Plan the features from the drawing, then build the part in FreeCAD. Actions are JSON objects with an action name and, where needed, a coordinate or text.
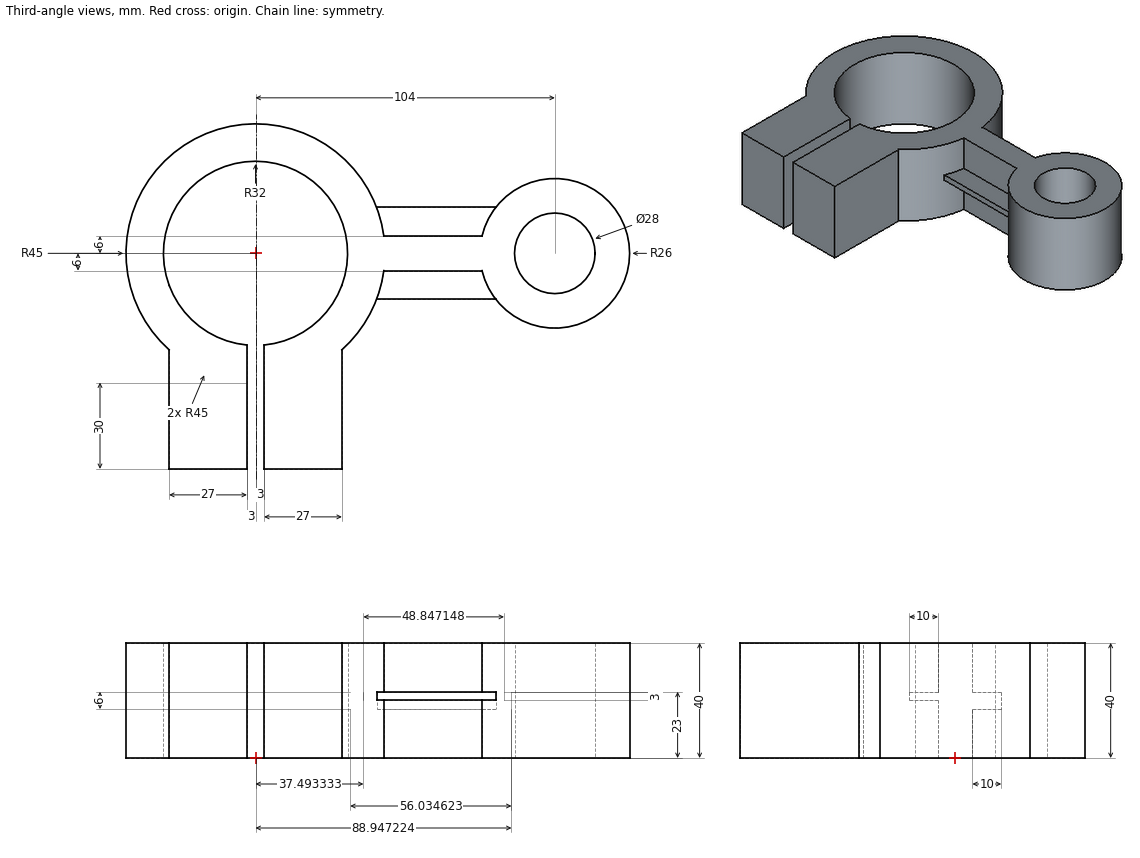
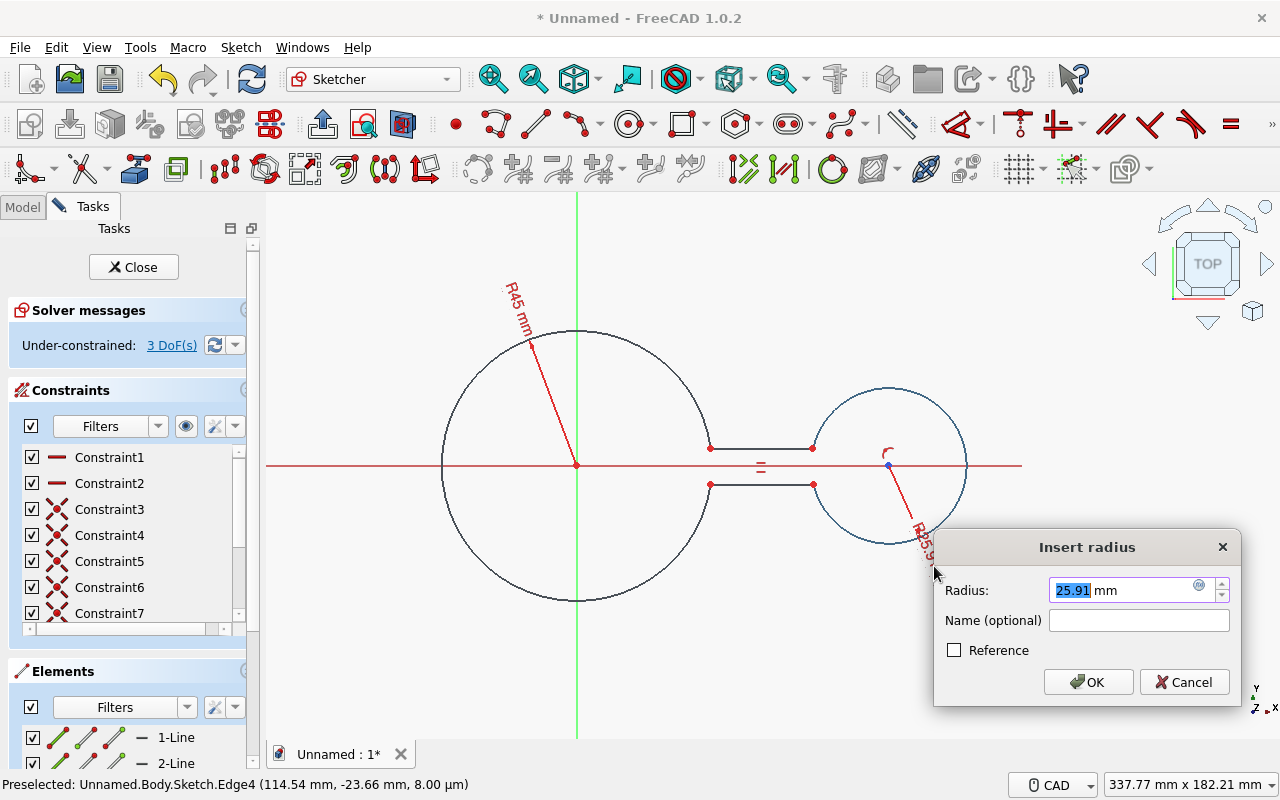
{"action": "type", "text": "26"}
{"action": "key", "text": "Return"}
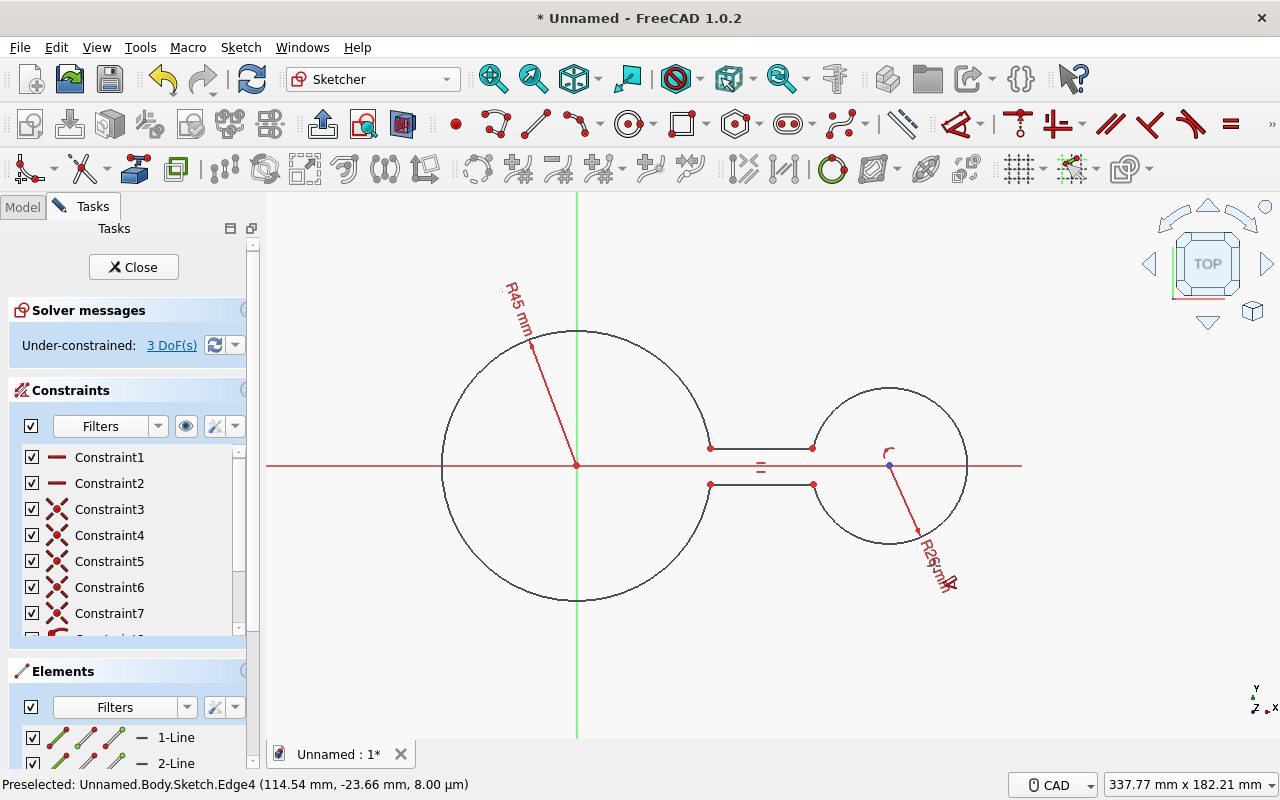
{"action": "scroll", "coordinate": [813, 449], "scroll_direction": "up", "scroll_amount": 4}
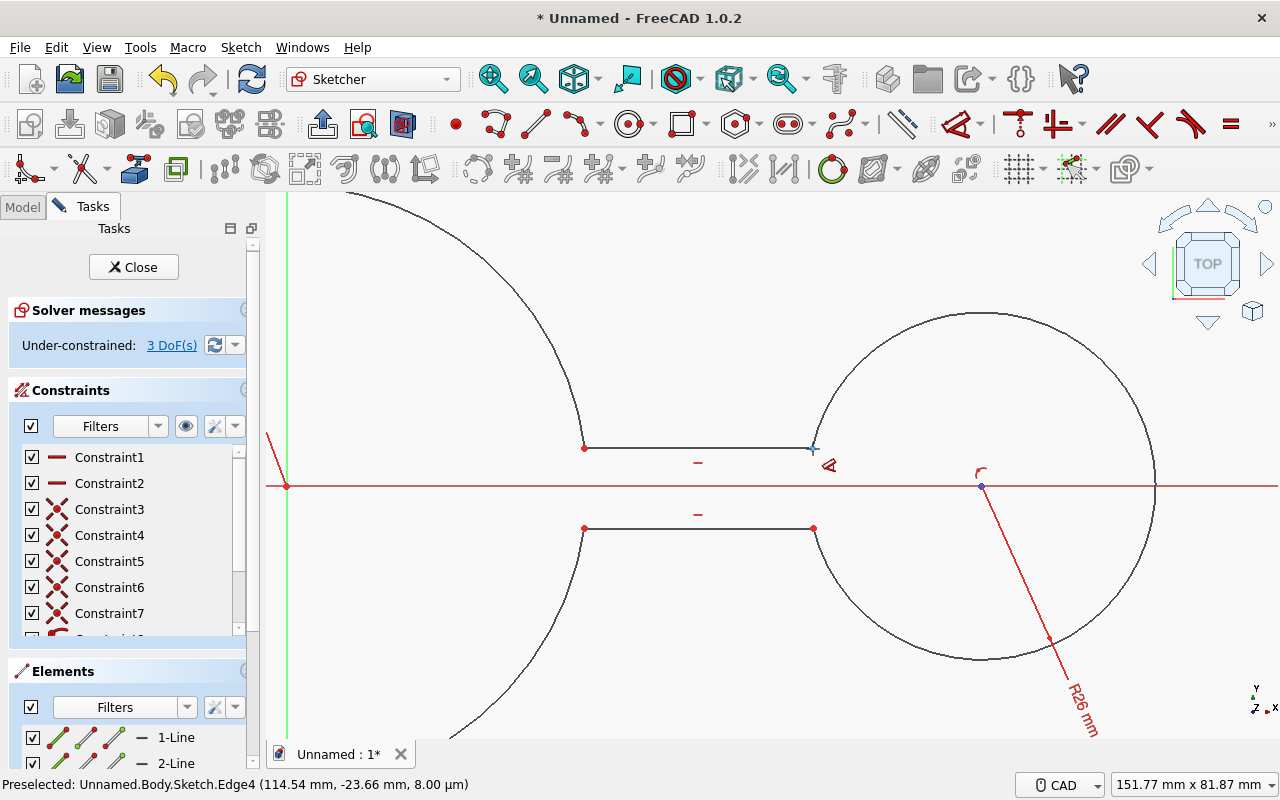
{"action": "left_click", "coordinate": [812, 448]}
{"action": "left_click", "coordinate": [846, 467]}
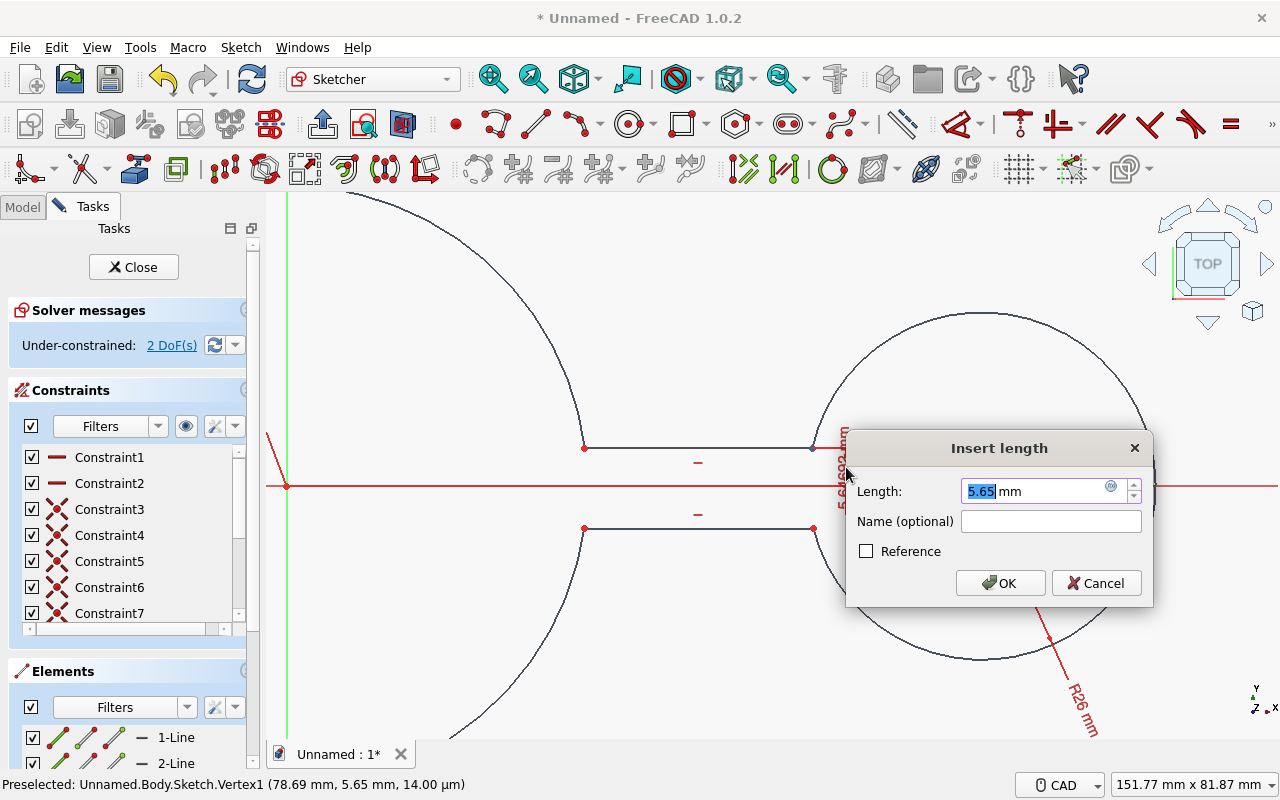
{"action": "type", "text": "6"}
{"action": "key", "text": "Return"}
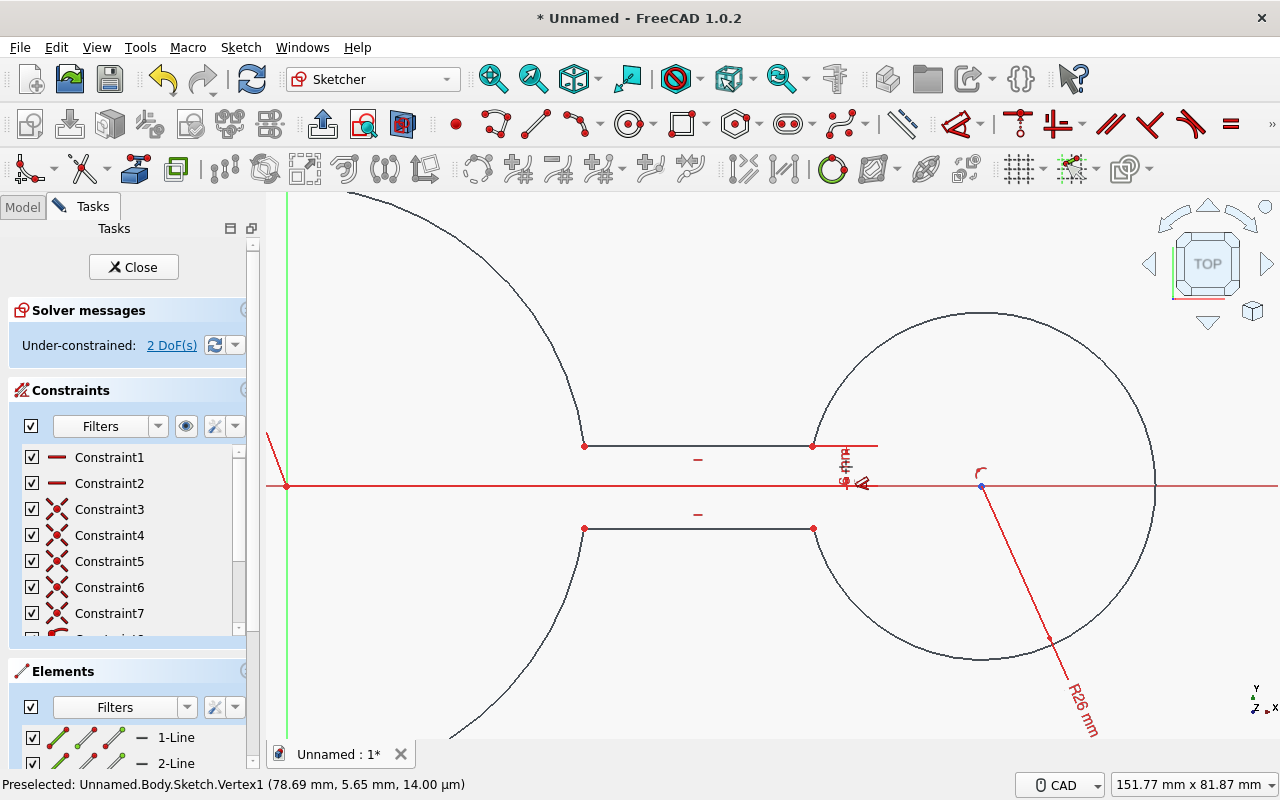
{"action": "left_click", "coordinate": [584, 529]}
{"action": "left_click", "coordinate": [618, 507]}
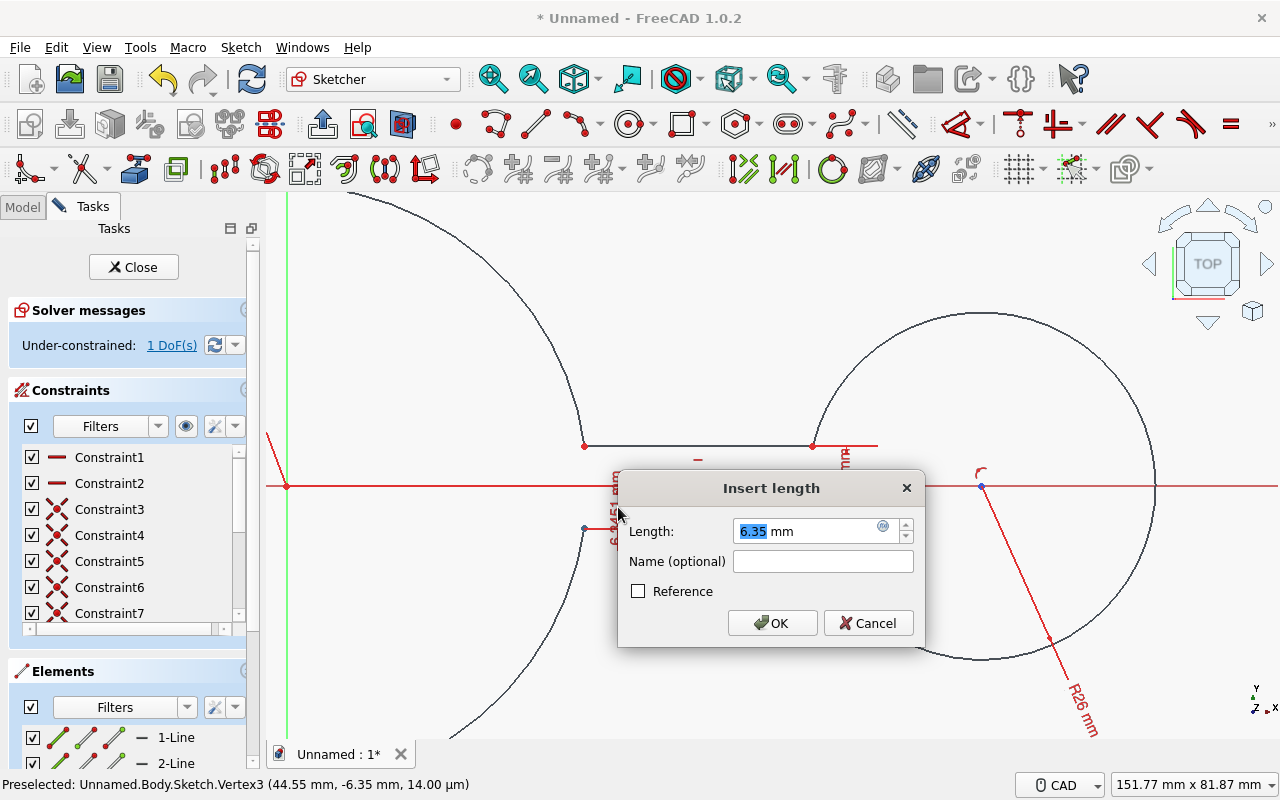
{"action": "type", "text": "6"}
{"action": "key", "text": "Return"}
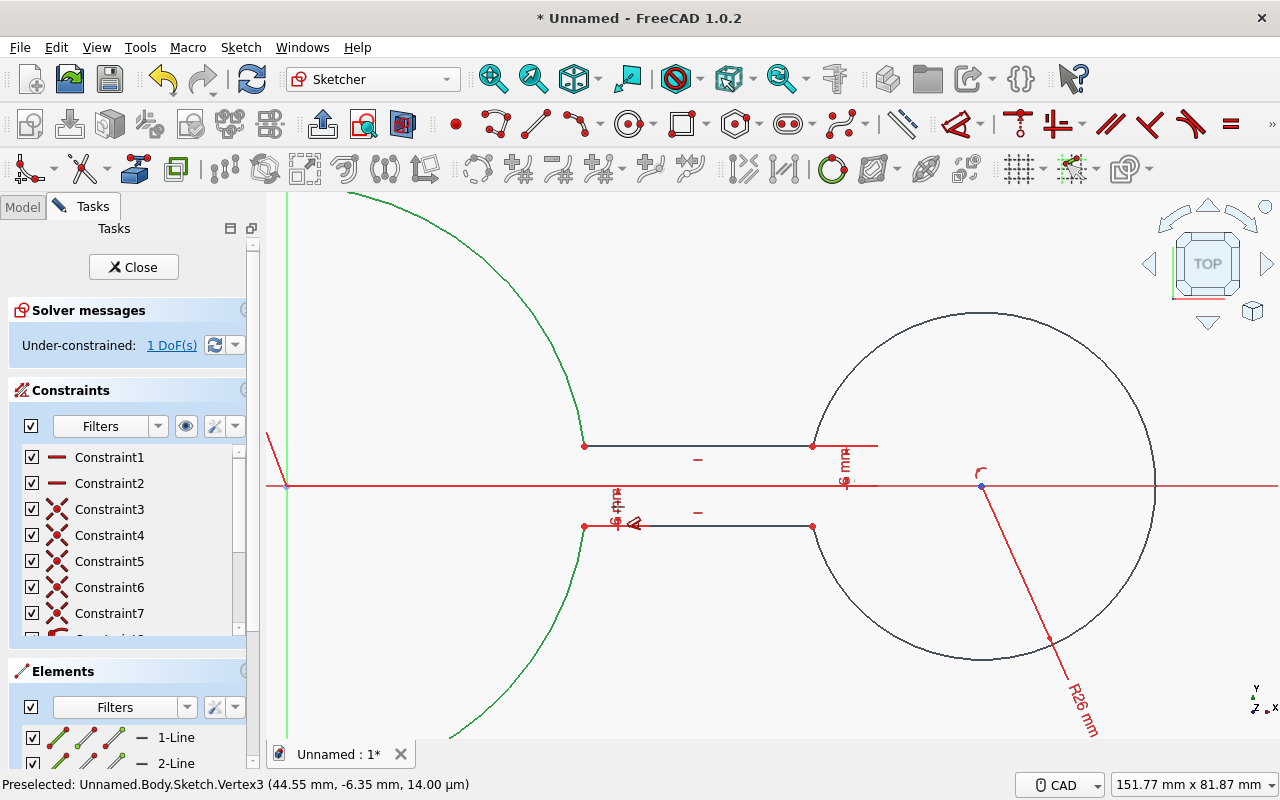
{"action": "left_click", "coordinate": [982, 486]}
{"action": "left_click", "coordinate": [480, 520]}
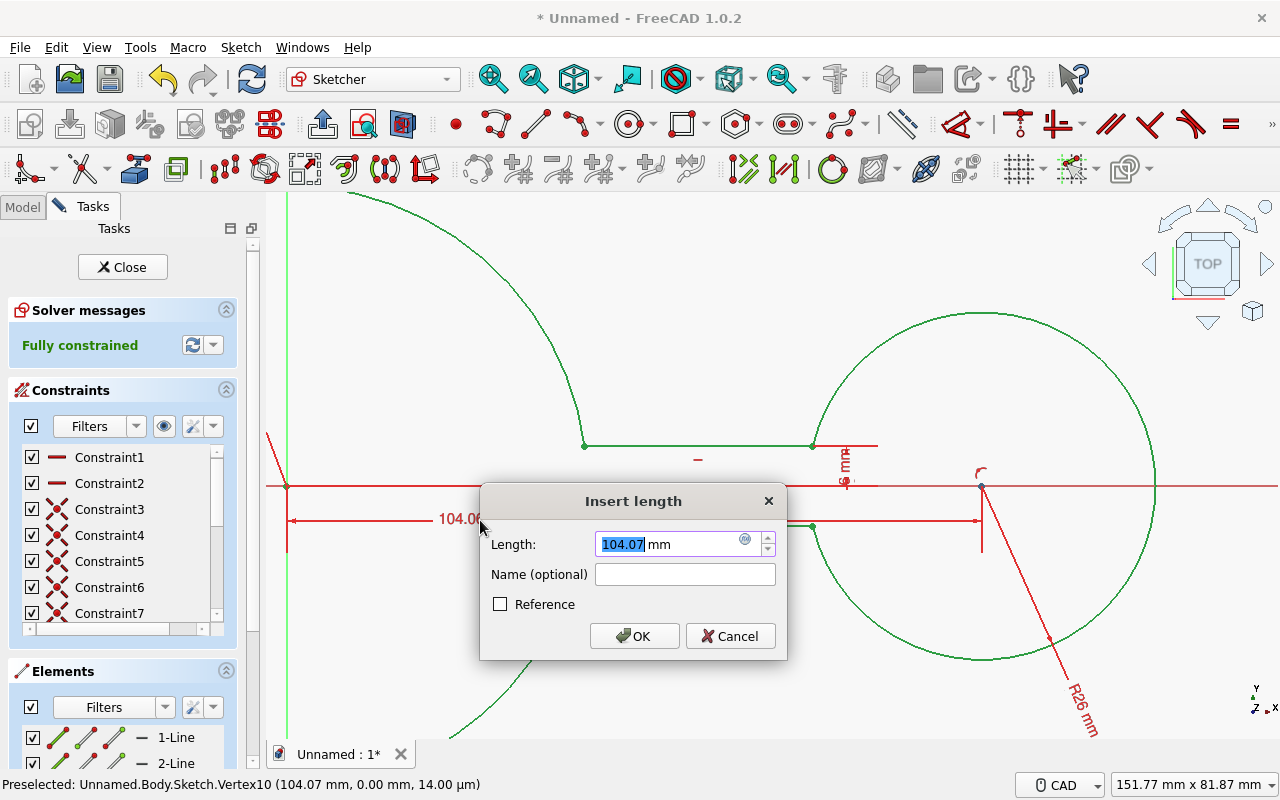
{"action": "type", "text": "104"}
{"action": "key", "text": "Return"}
{"action": "key", "text": "Escape"}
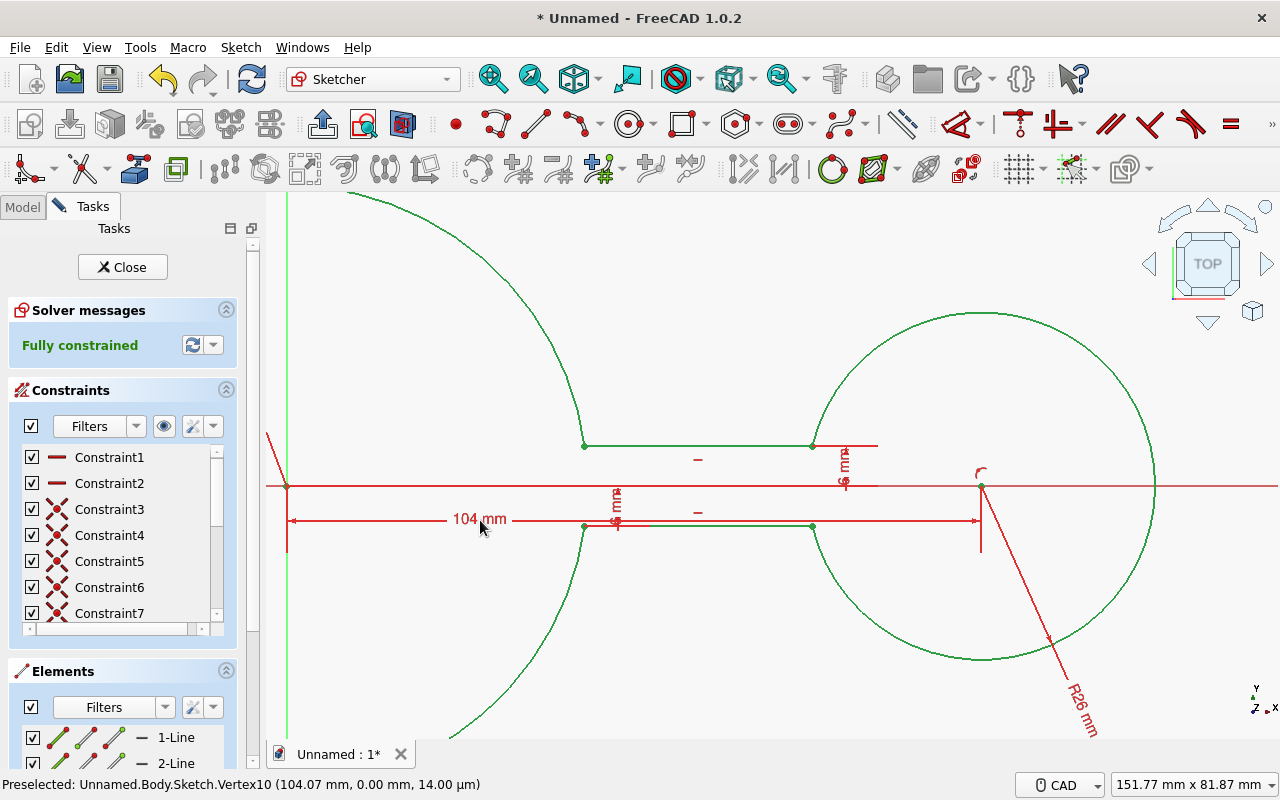
{"action": "left_click", "coordinate": [123, 267]}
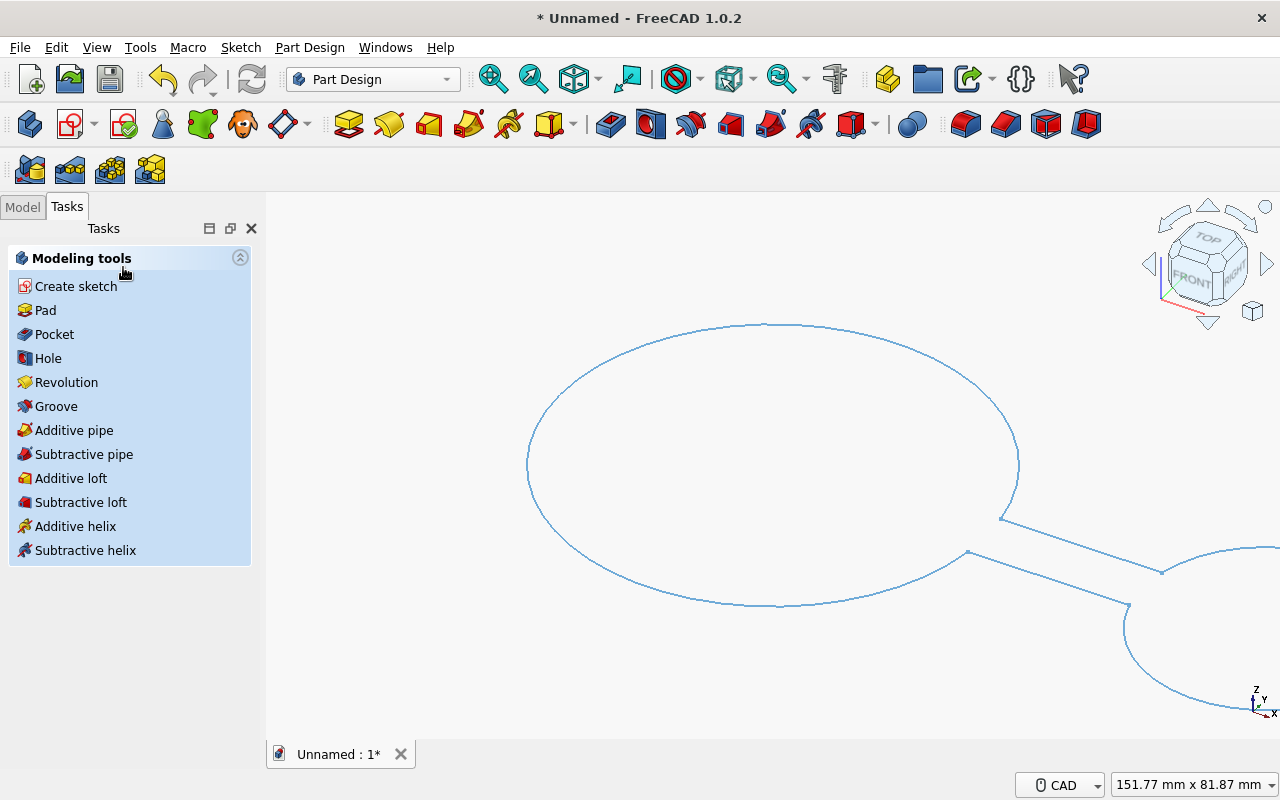
{"action": "left_click", "coordinate": [350, 124]}